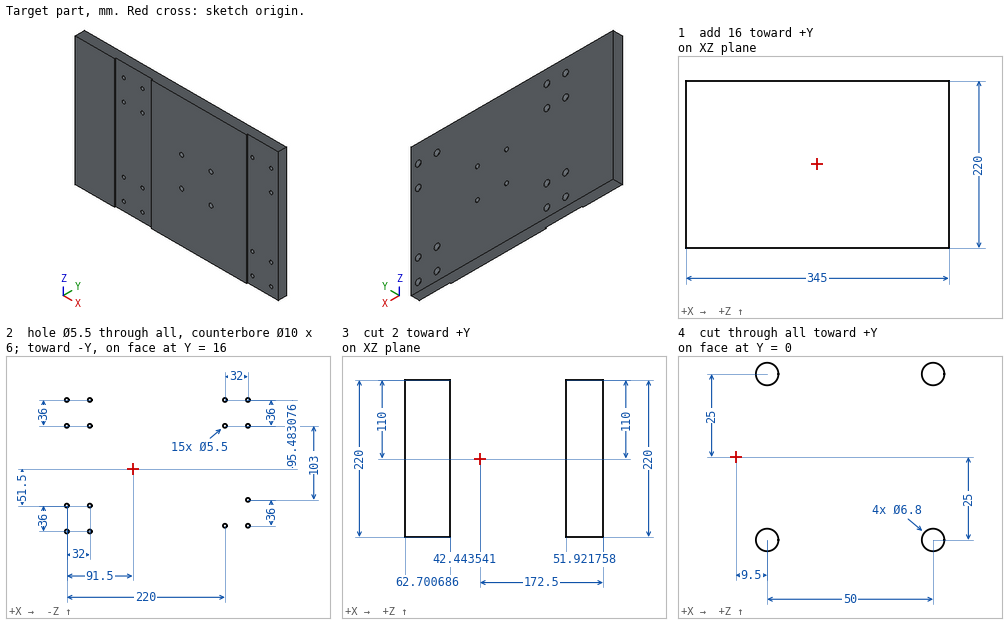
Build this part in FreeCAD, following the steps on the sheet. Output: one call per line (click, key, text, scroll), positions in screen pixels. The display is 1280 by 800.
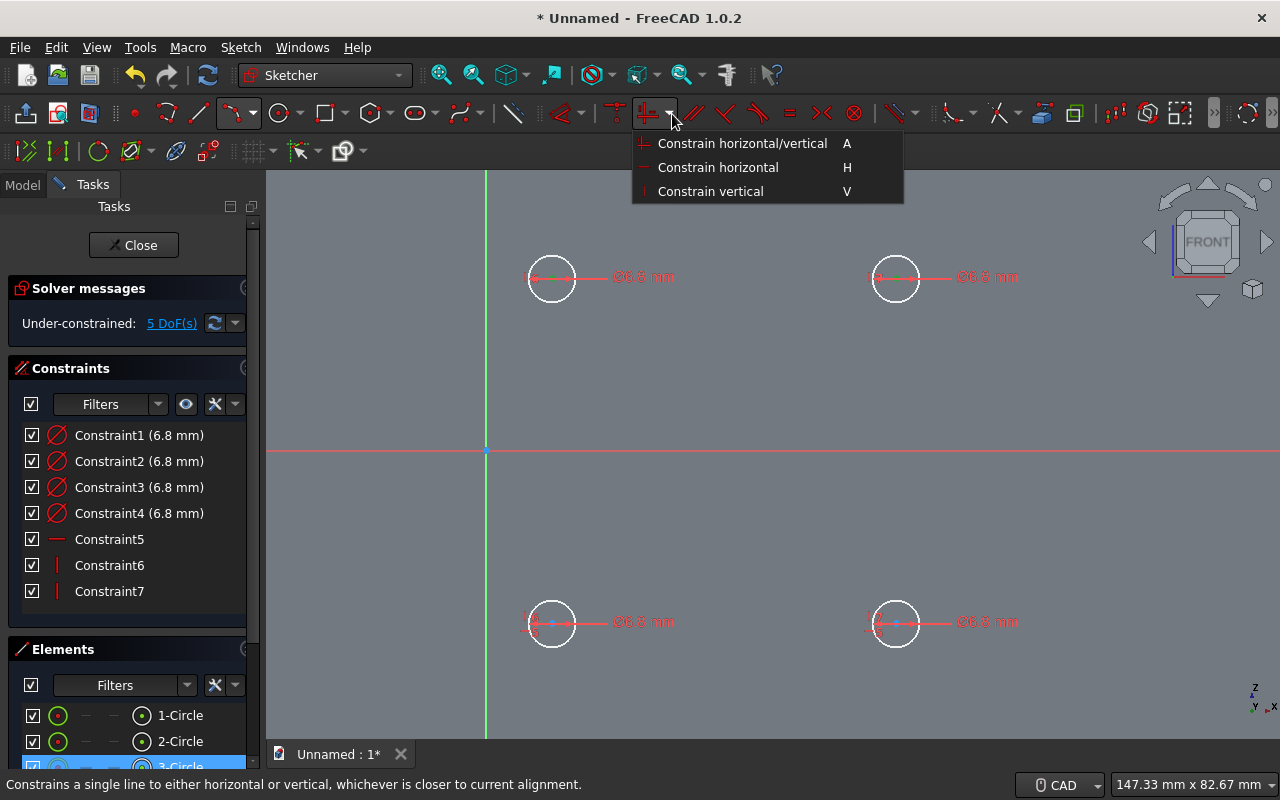
click(768, 167)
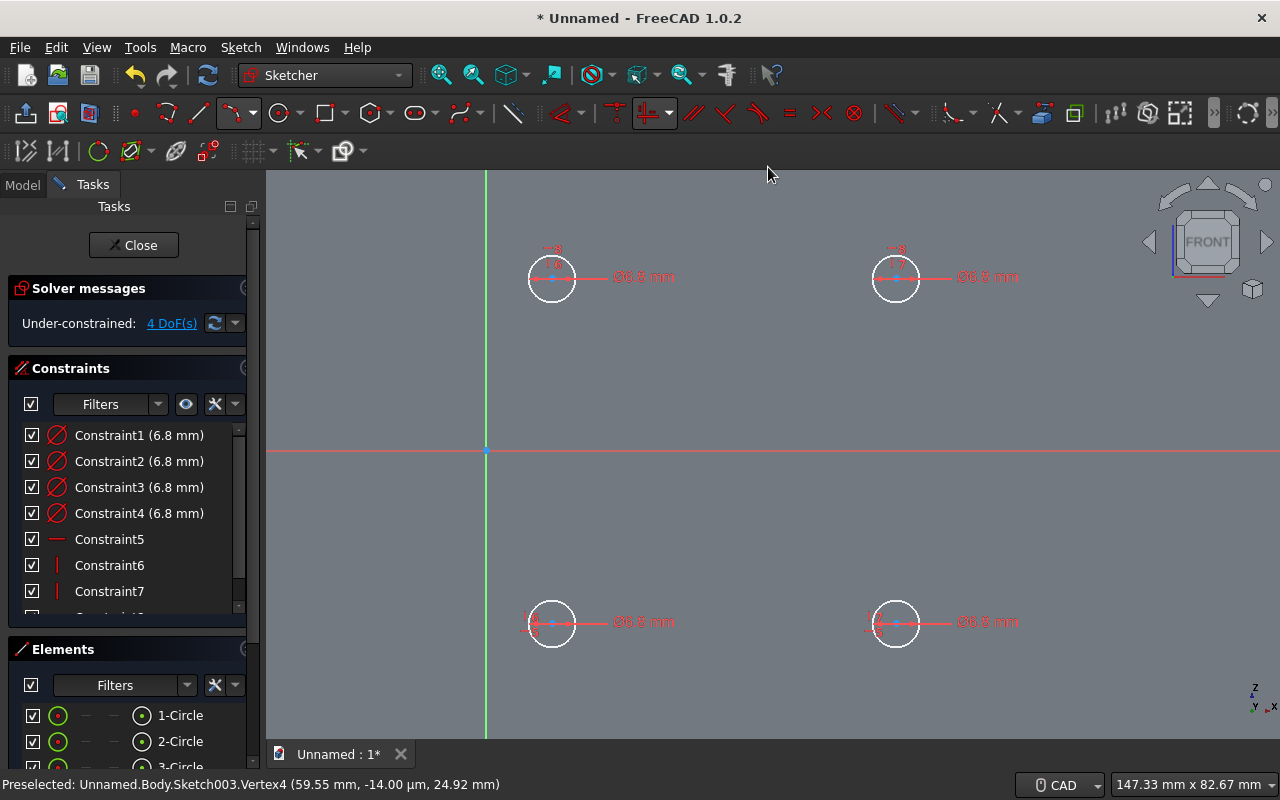
key(d)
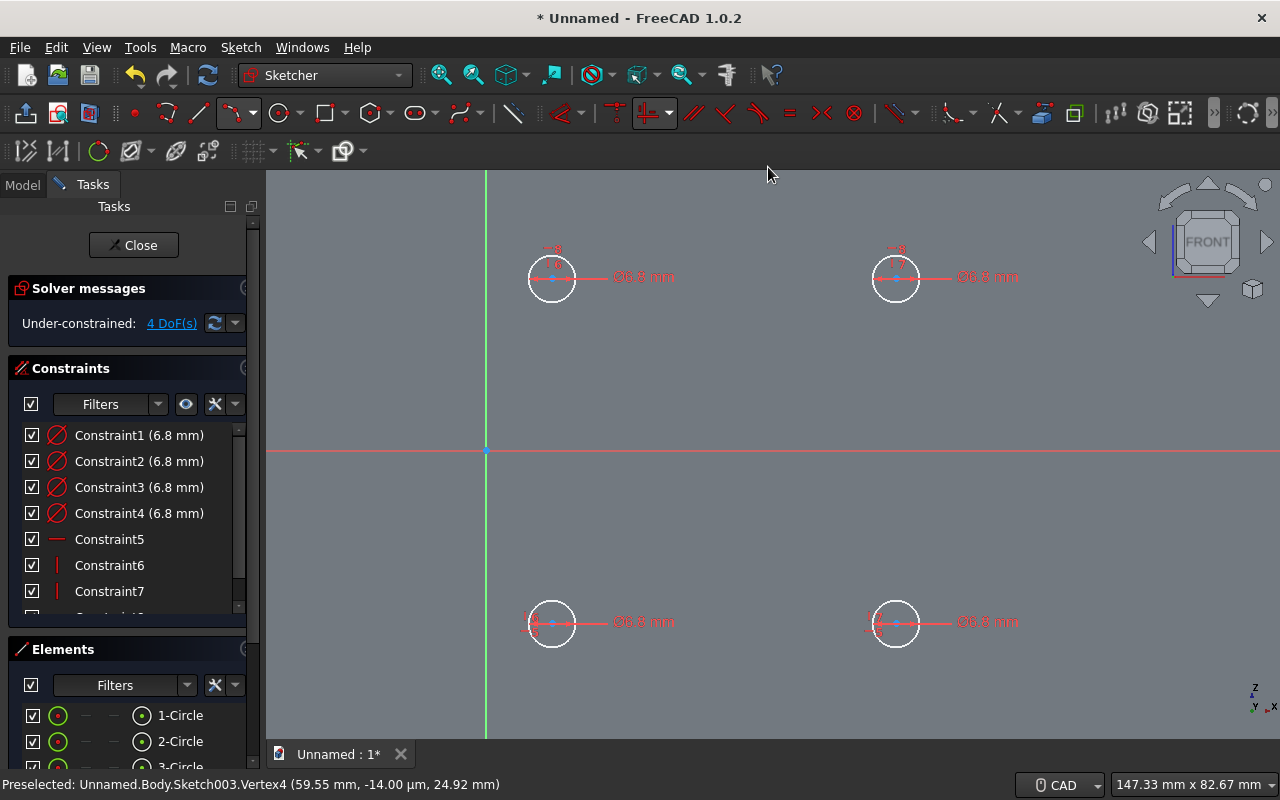
click(896, 624)
click(452, 537)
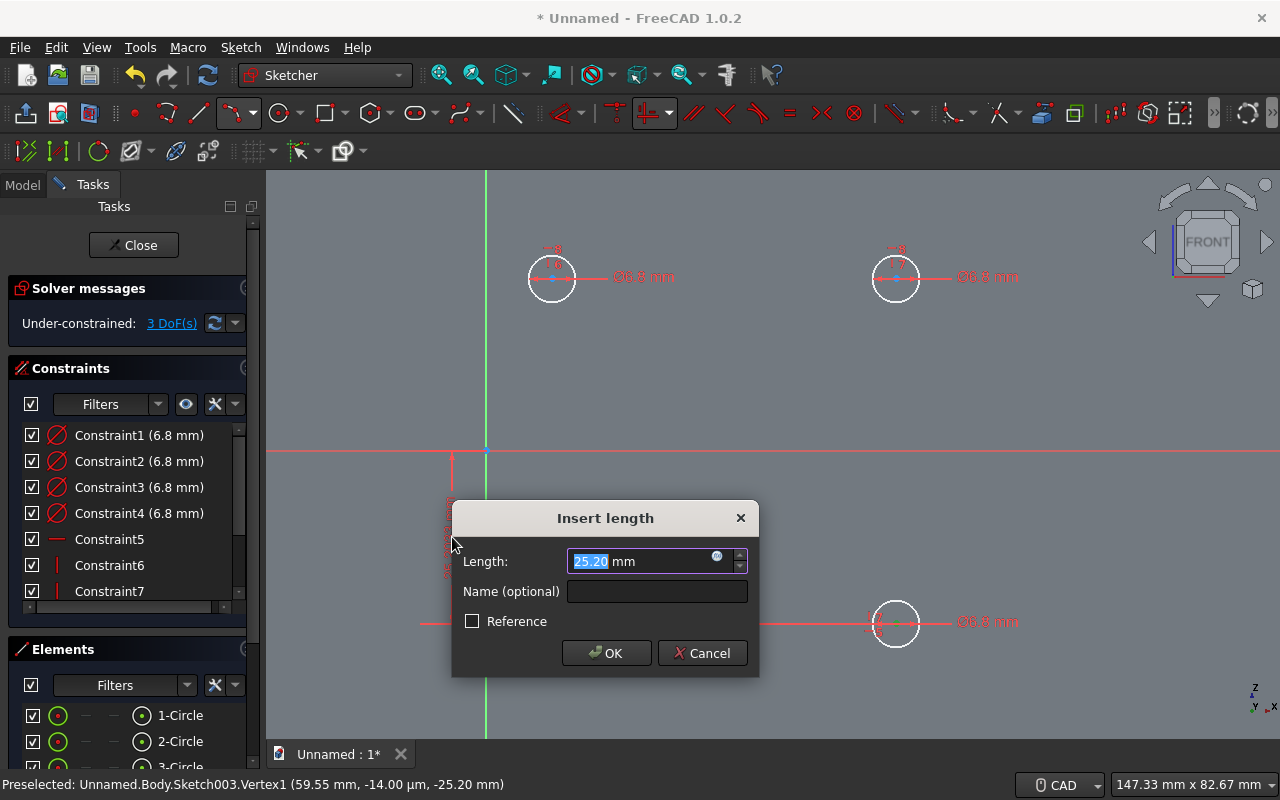
text(25)
key(Return)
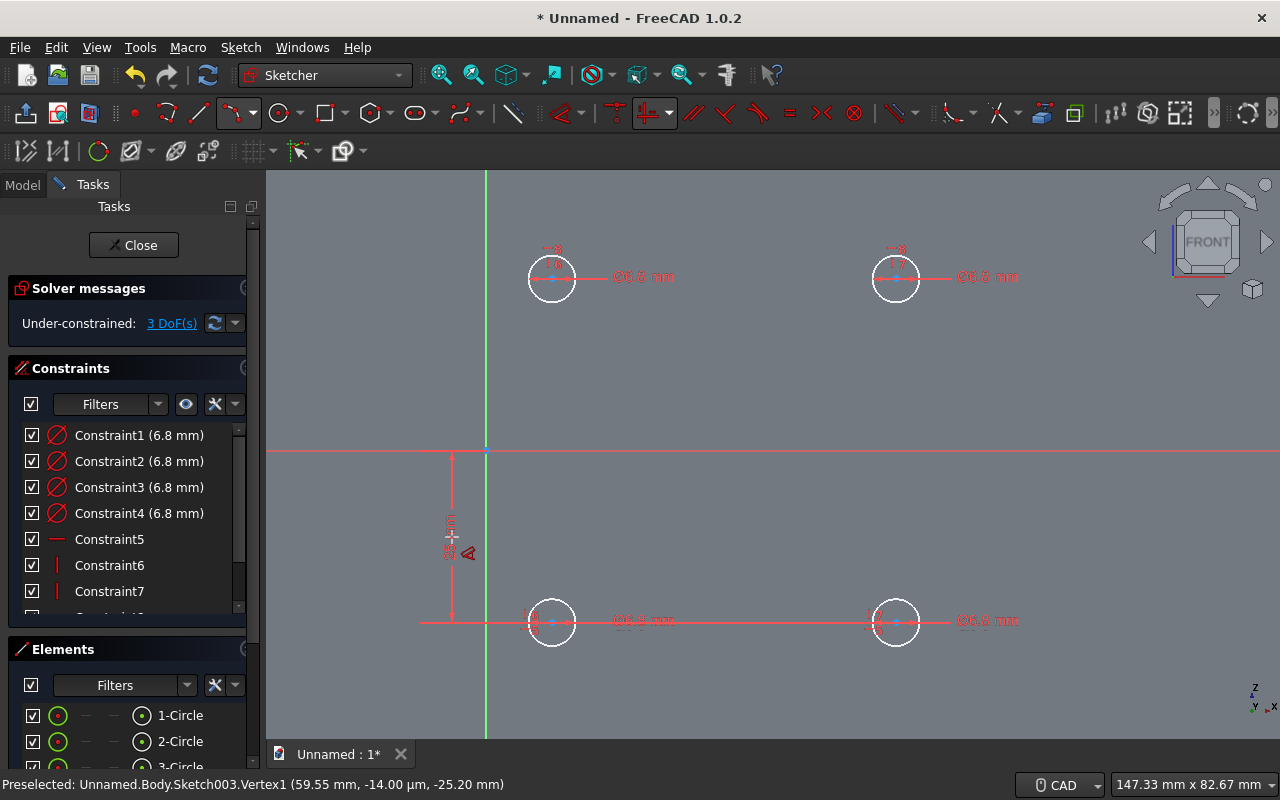
click(552, 279)
click(452, 365)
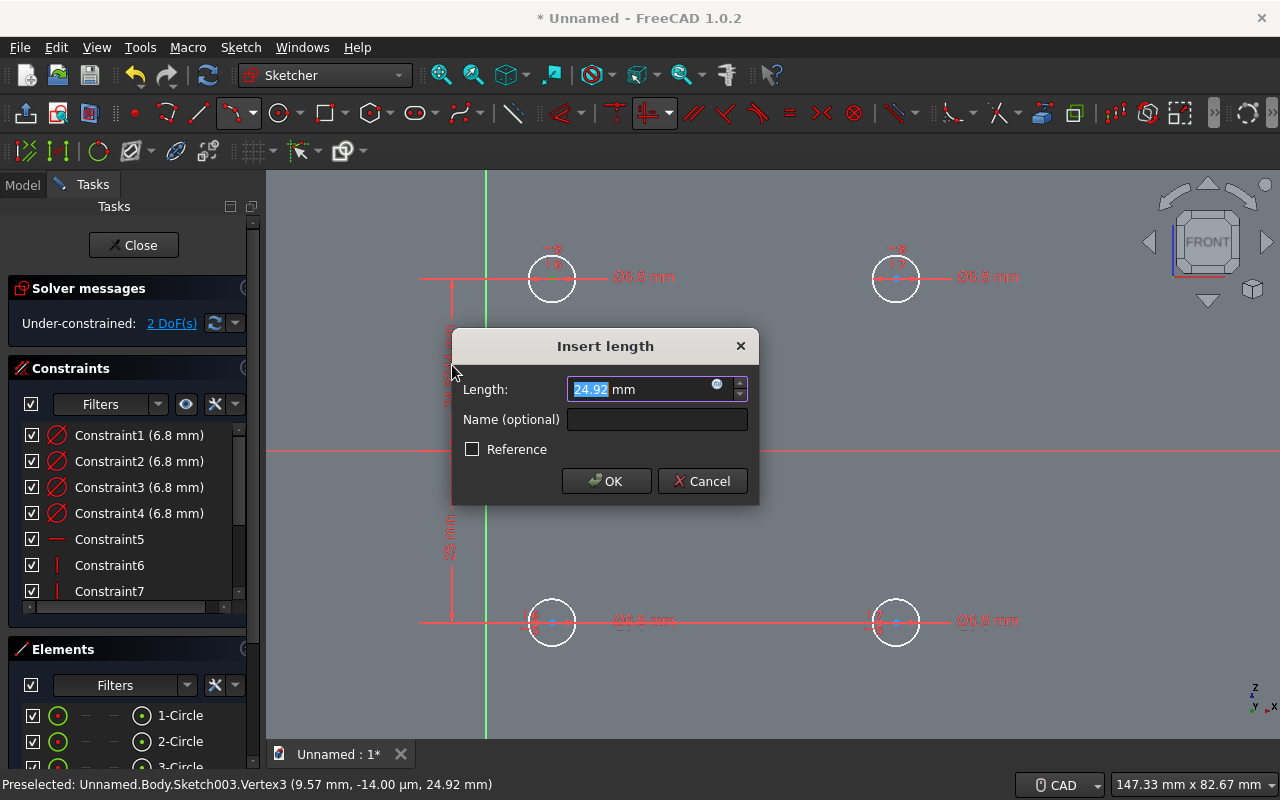
text(25)
key(Return)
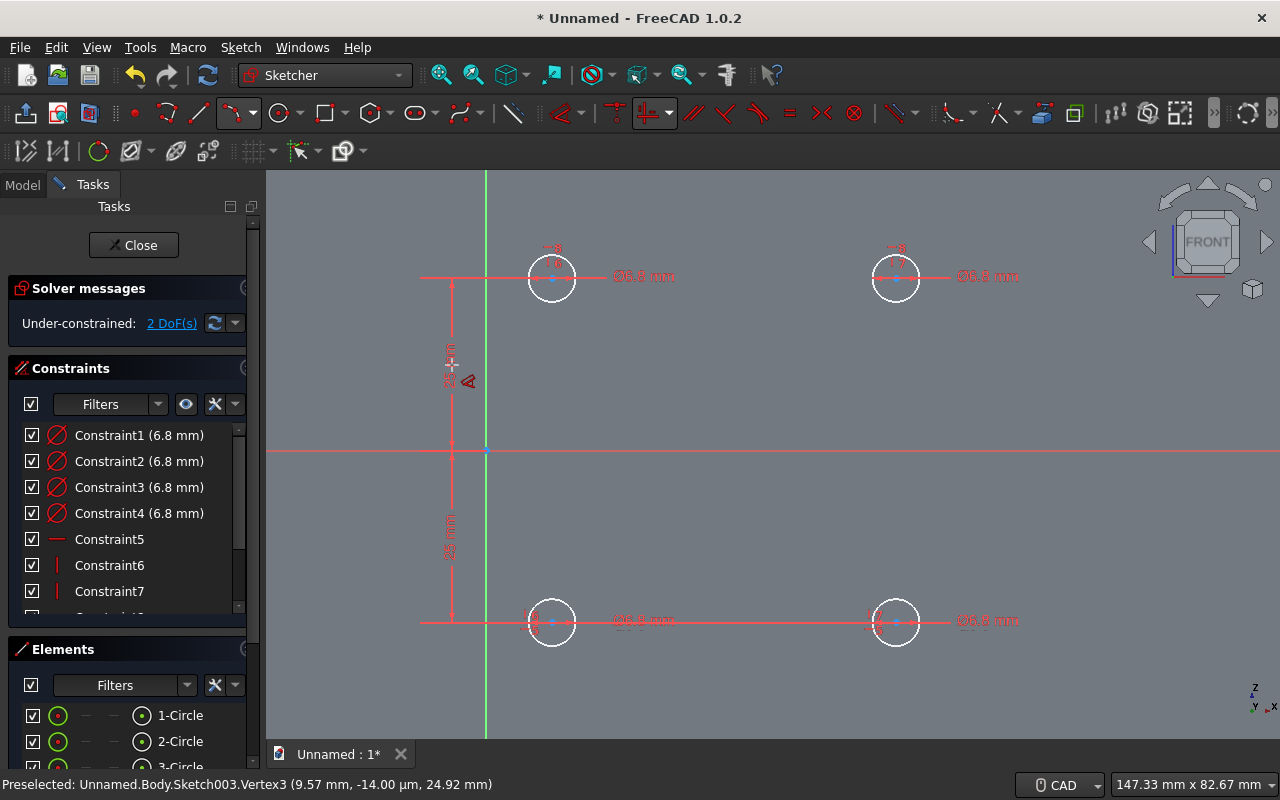
click(552, 623)
click(519, 657)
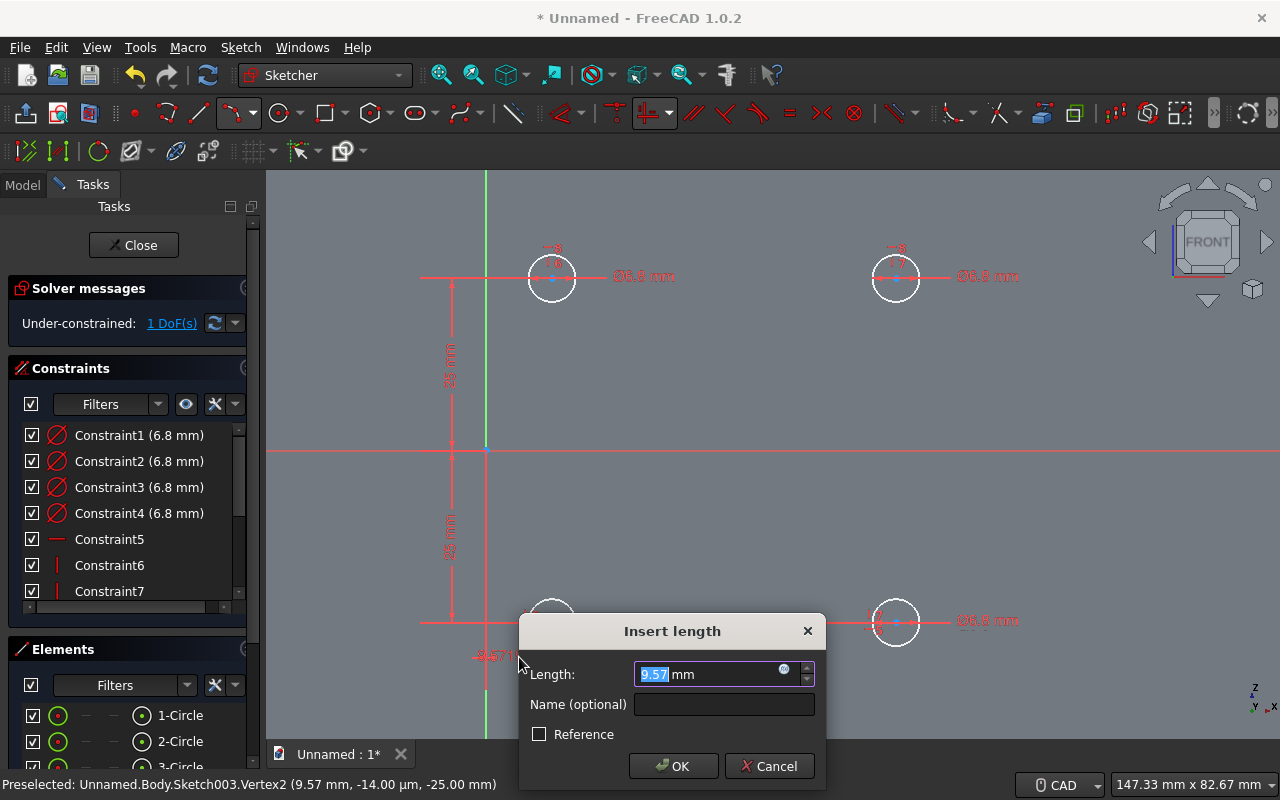
text(9.5)
key(Return)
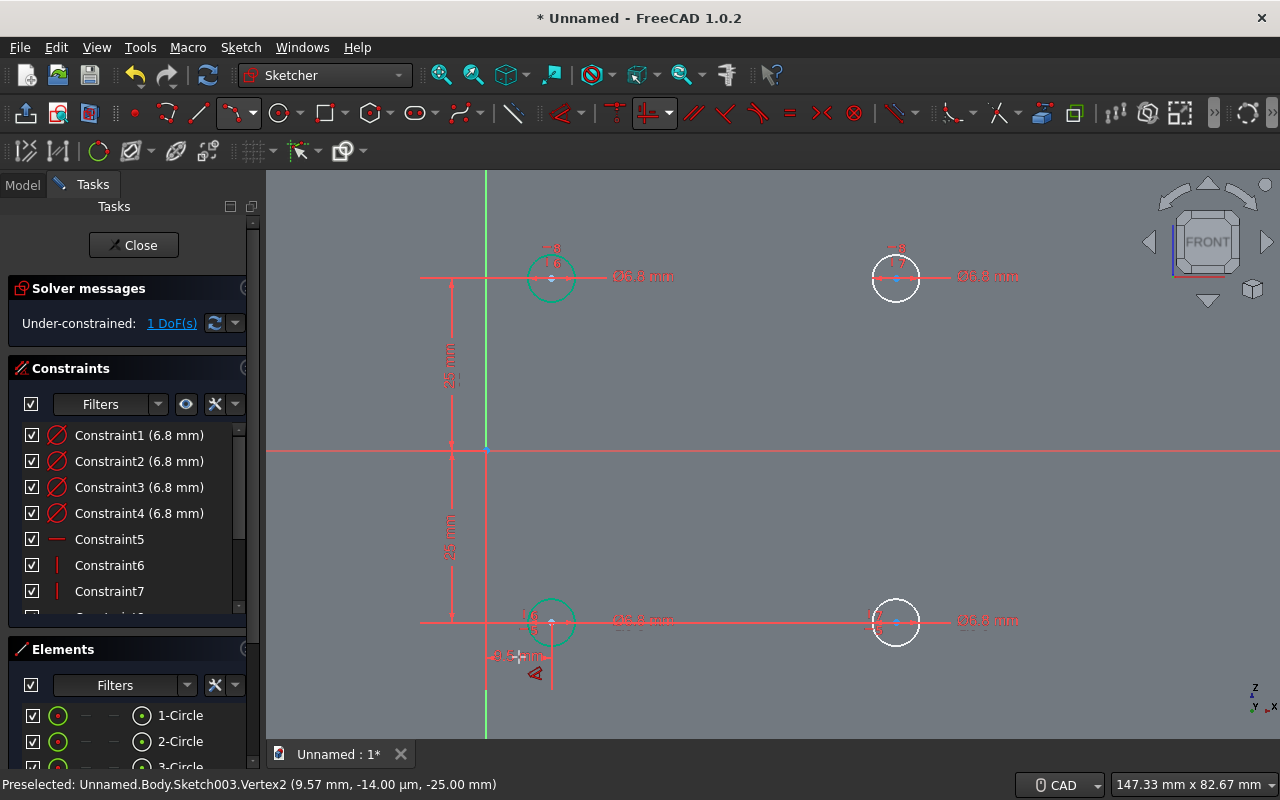
click(896, 623)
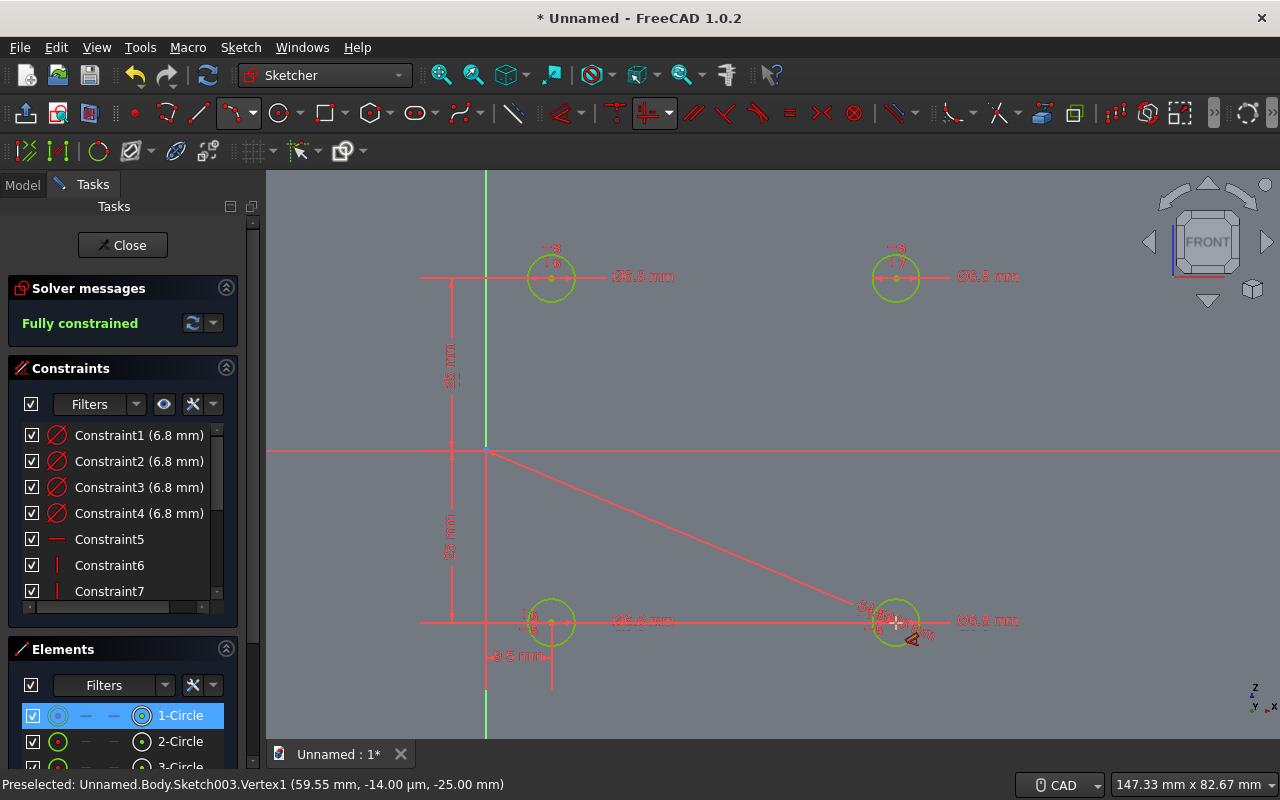
click(552, 623)
click(724, 657)